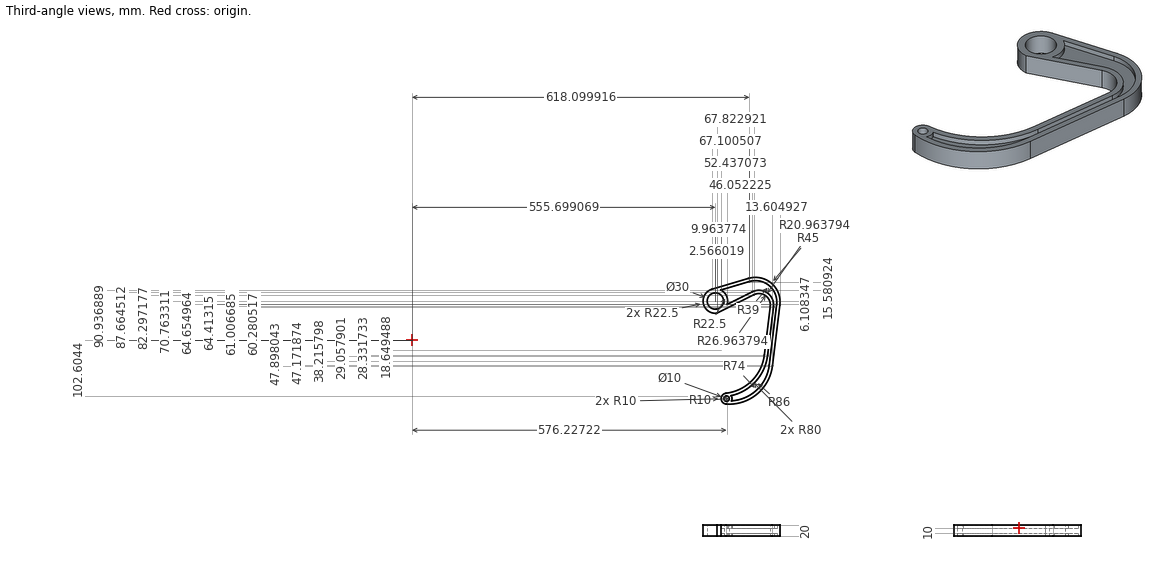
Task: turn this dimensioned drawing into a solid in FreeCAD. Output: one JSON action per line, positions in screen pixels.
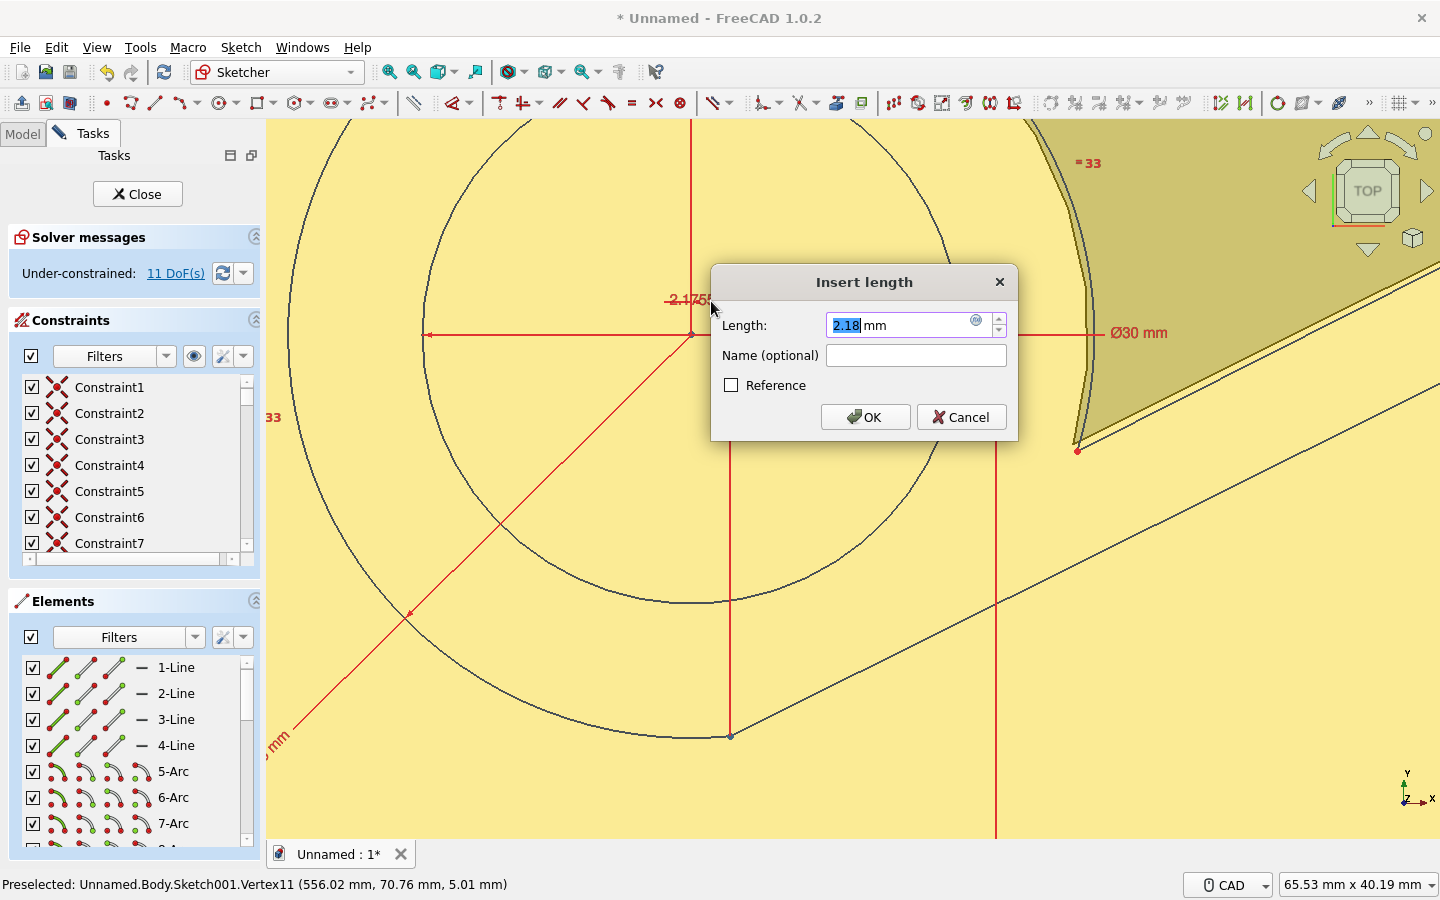
{"action": "type", "text": "2.566019"}
{"action": "key", "text": "Return"}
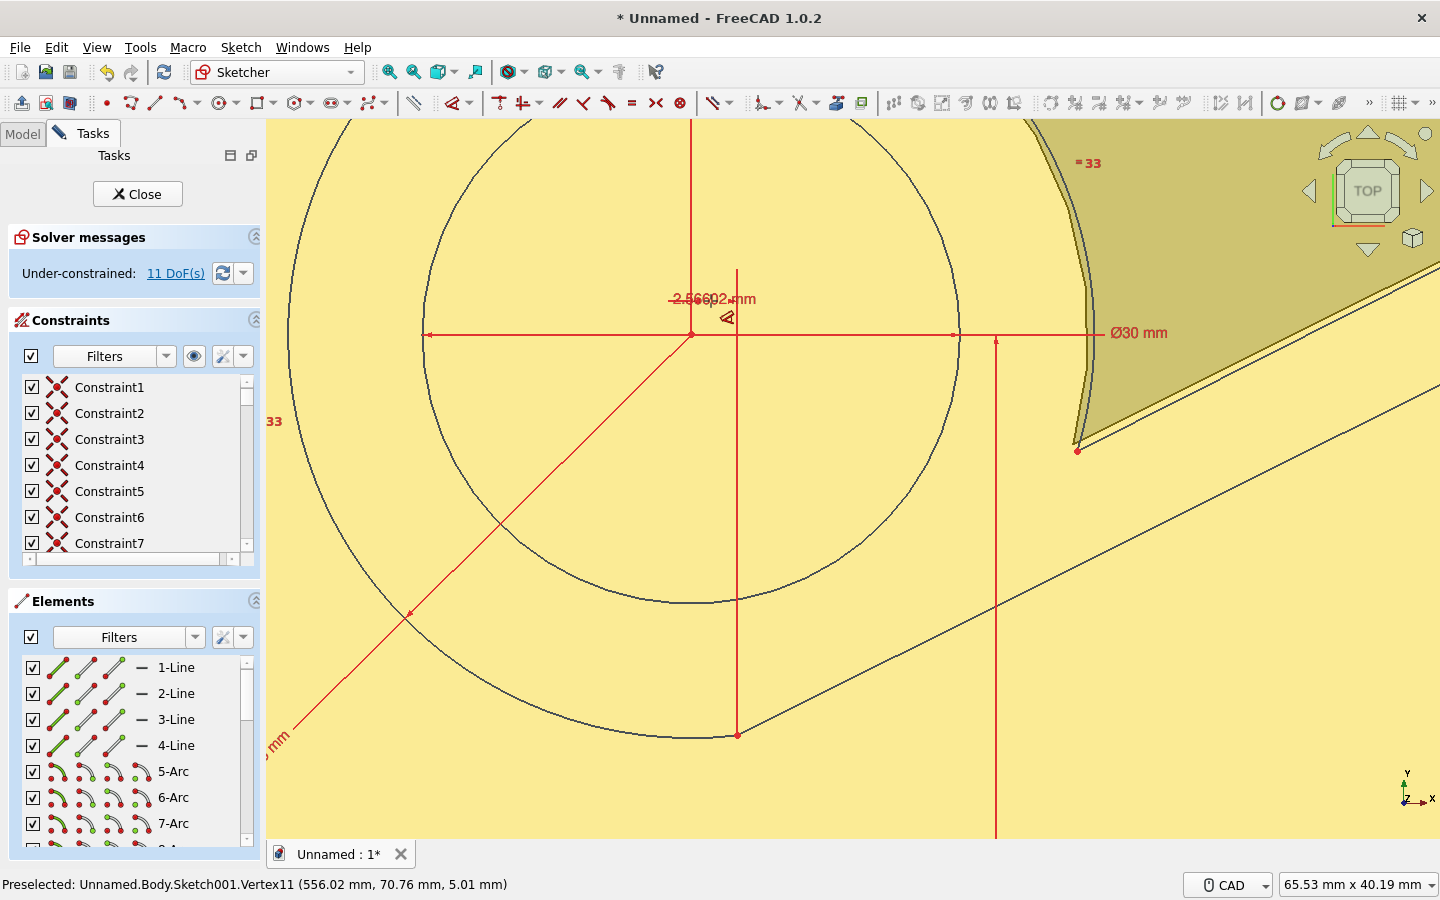
{"action": "left_click", "coordinate": [1077, 452]}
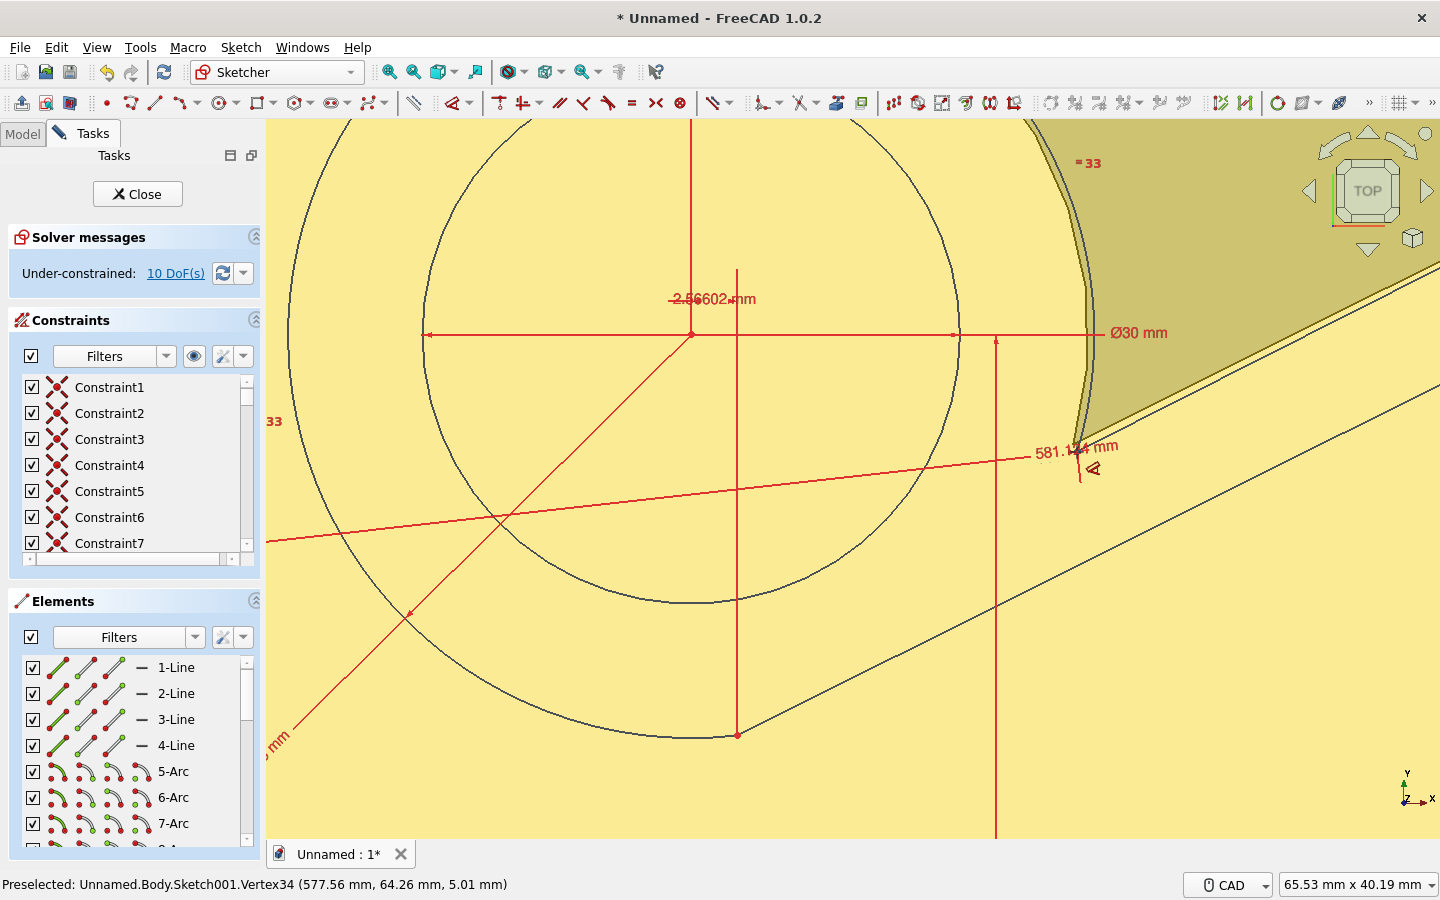
{"action": "left_click", "coordinate": [691, 335]}
{"action": "left_click", "coordinate": [657, 393]}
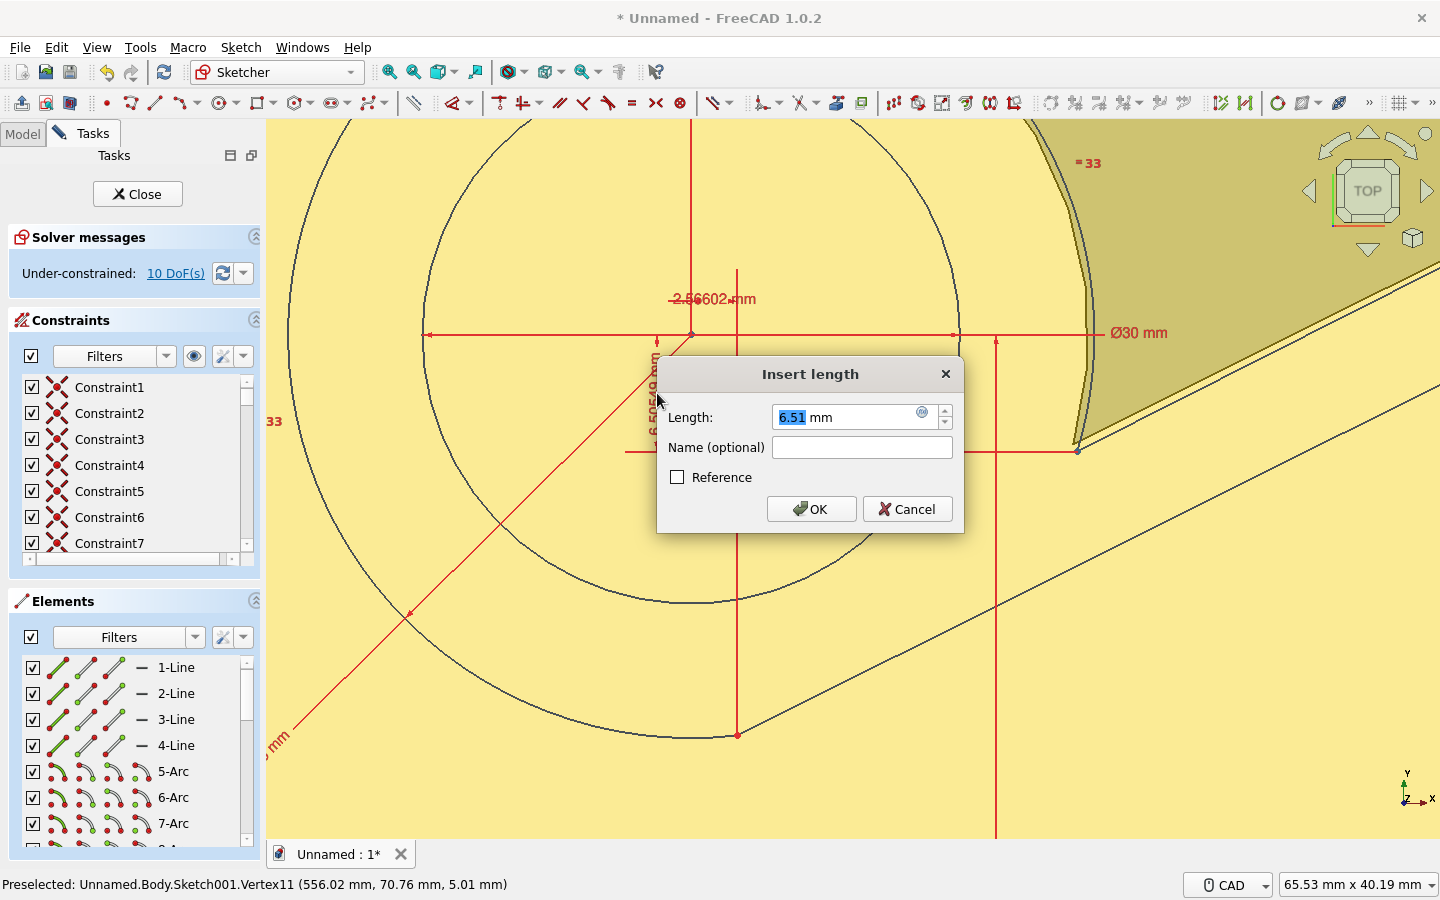
{"action": "type", "text": "6.108347"}
{"action": "key", "text": "Return"}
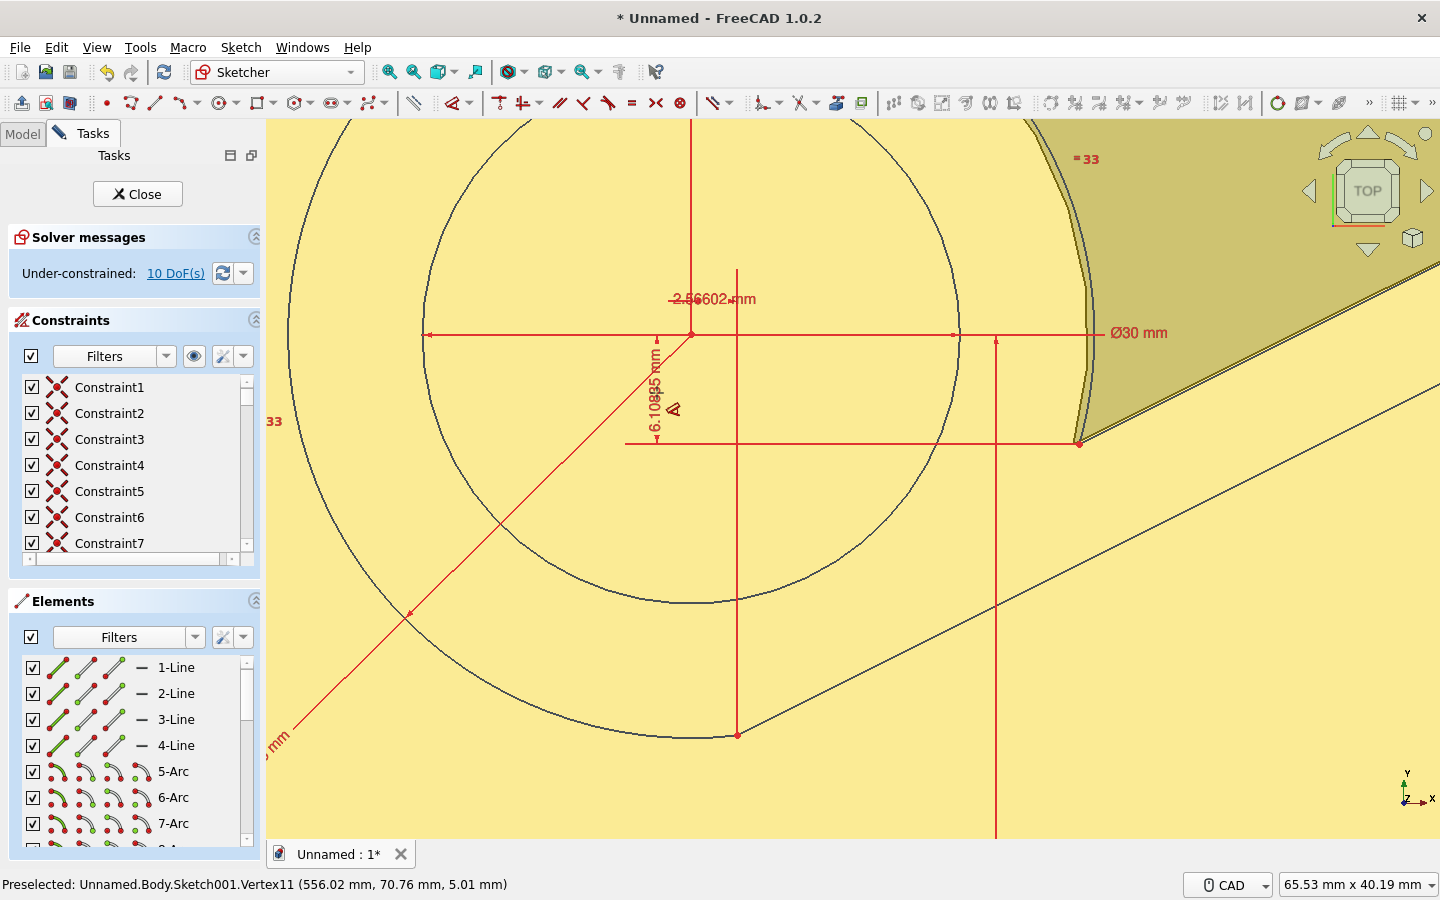
{"action": "scroll", "coordinate": [690, 333], "scroll_direction": "down", "scroll_amount": 11}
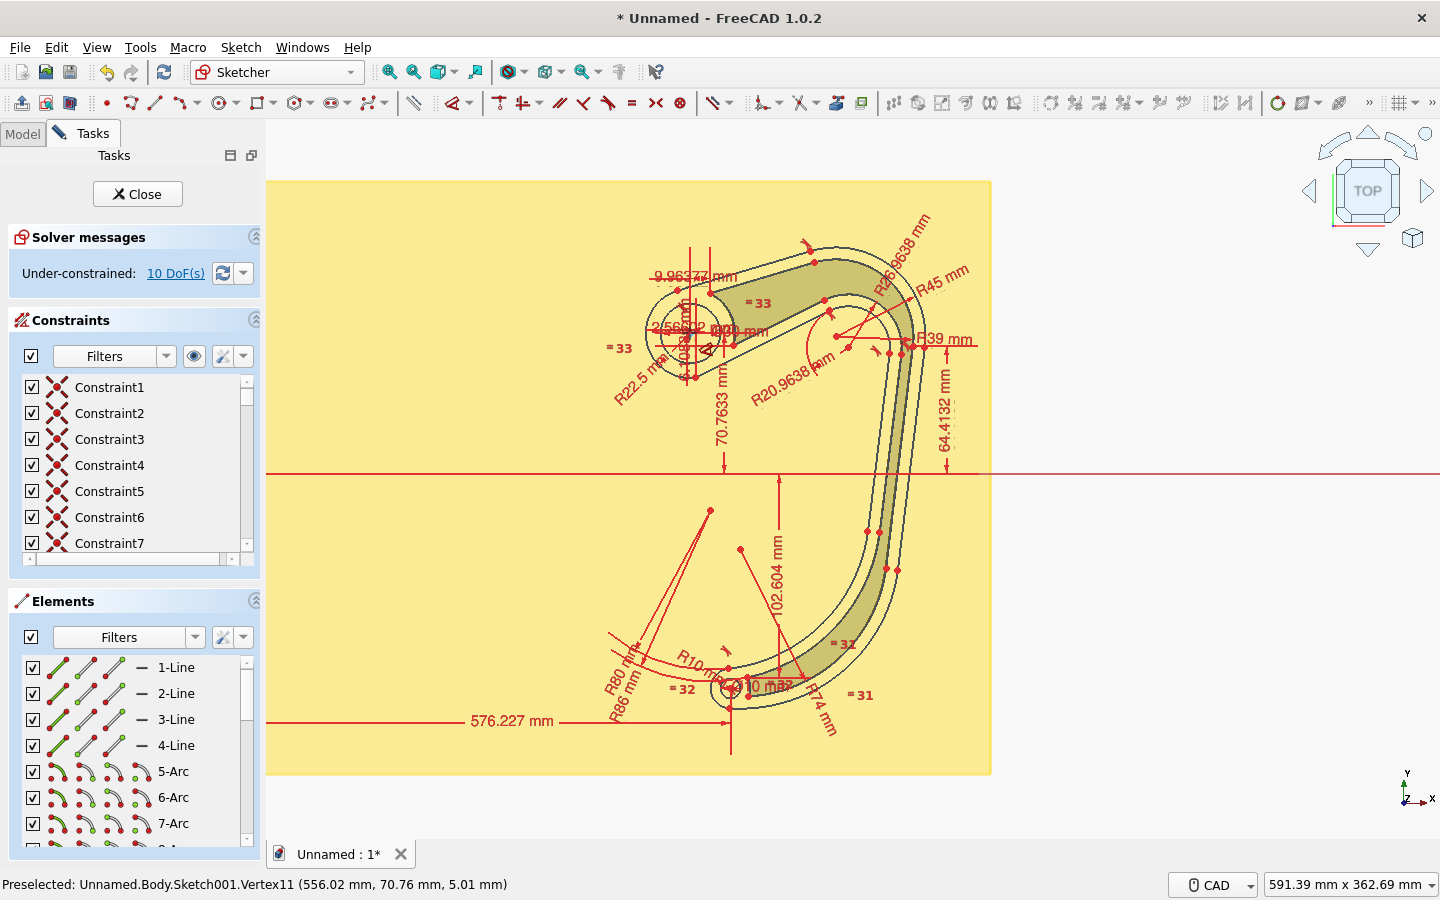
{"action": "left_click", "coordinate": [830, 311]}
{"action": "left_click", "coordinate": [864, 355]}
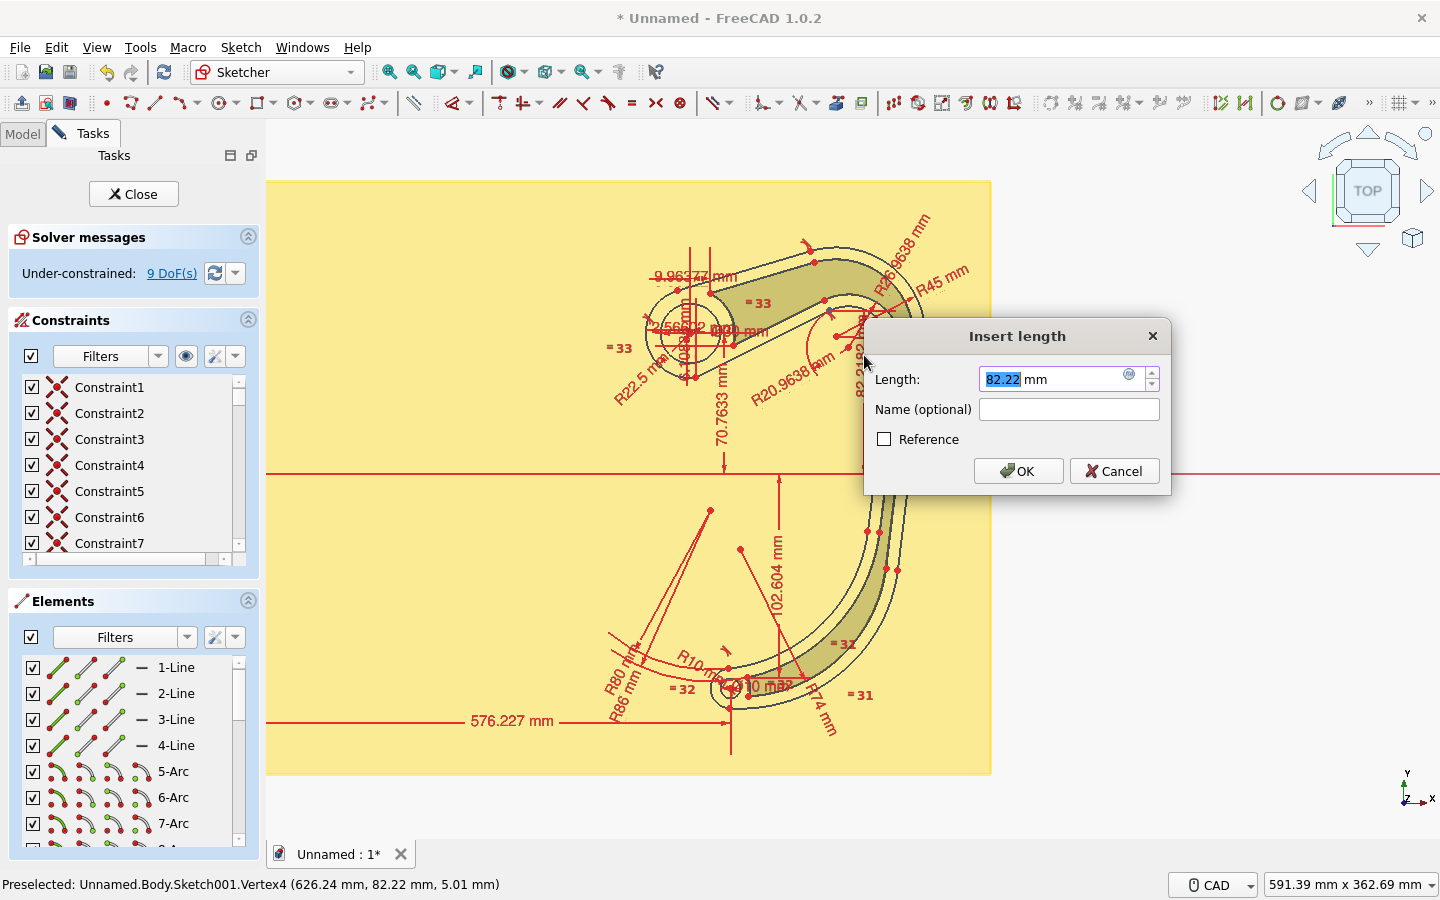
{"action": "type", "text": "82.297177"}
{"action": "key", "text": "Return"}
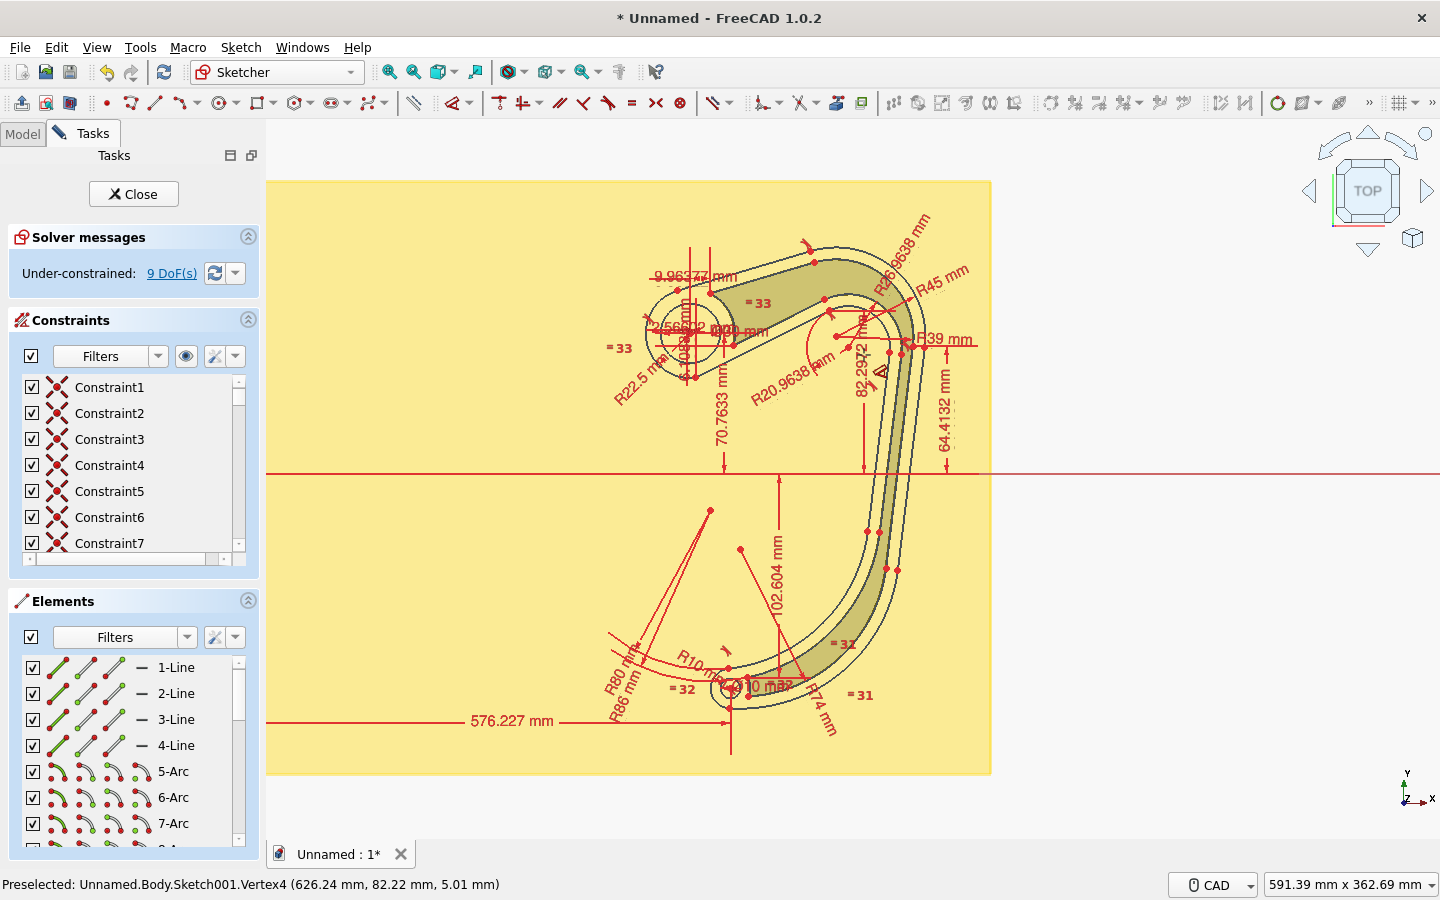
{"action": "left_click", "coordinate": [890, 353]}
{"action": "left_click", "coordinate": [948, 386]}